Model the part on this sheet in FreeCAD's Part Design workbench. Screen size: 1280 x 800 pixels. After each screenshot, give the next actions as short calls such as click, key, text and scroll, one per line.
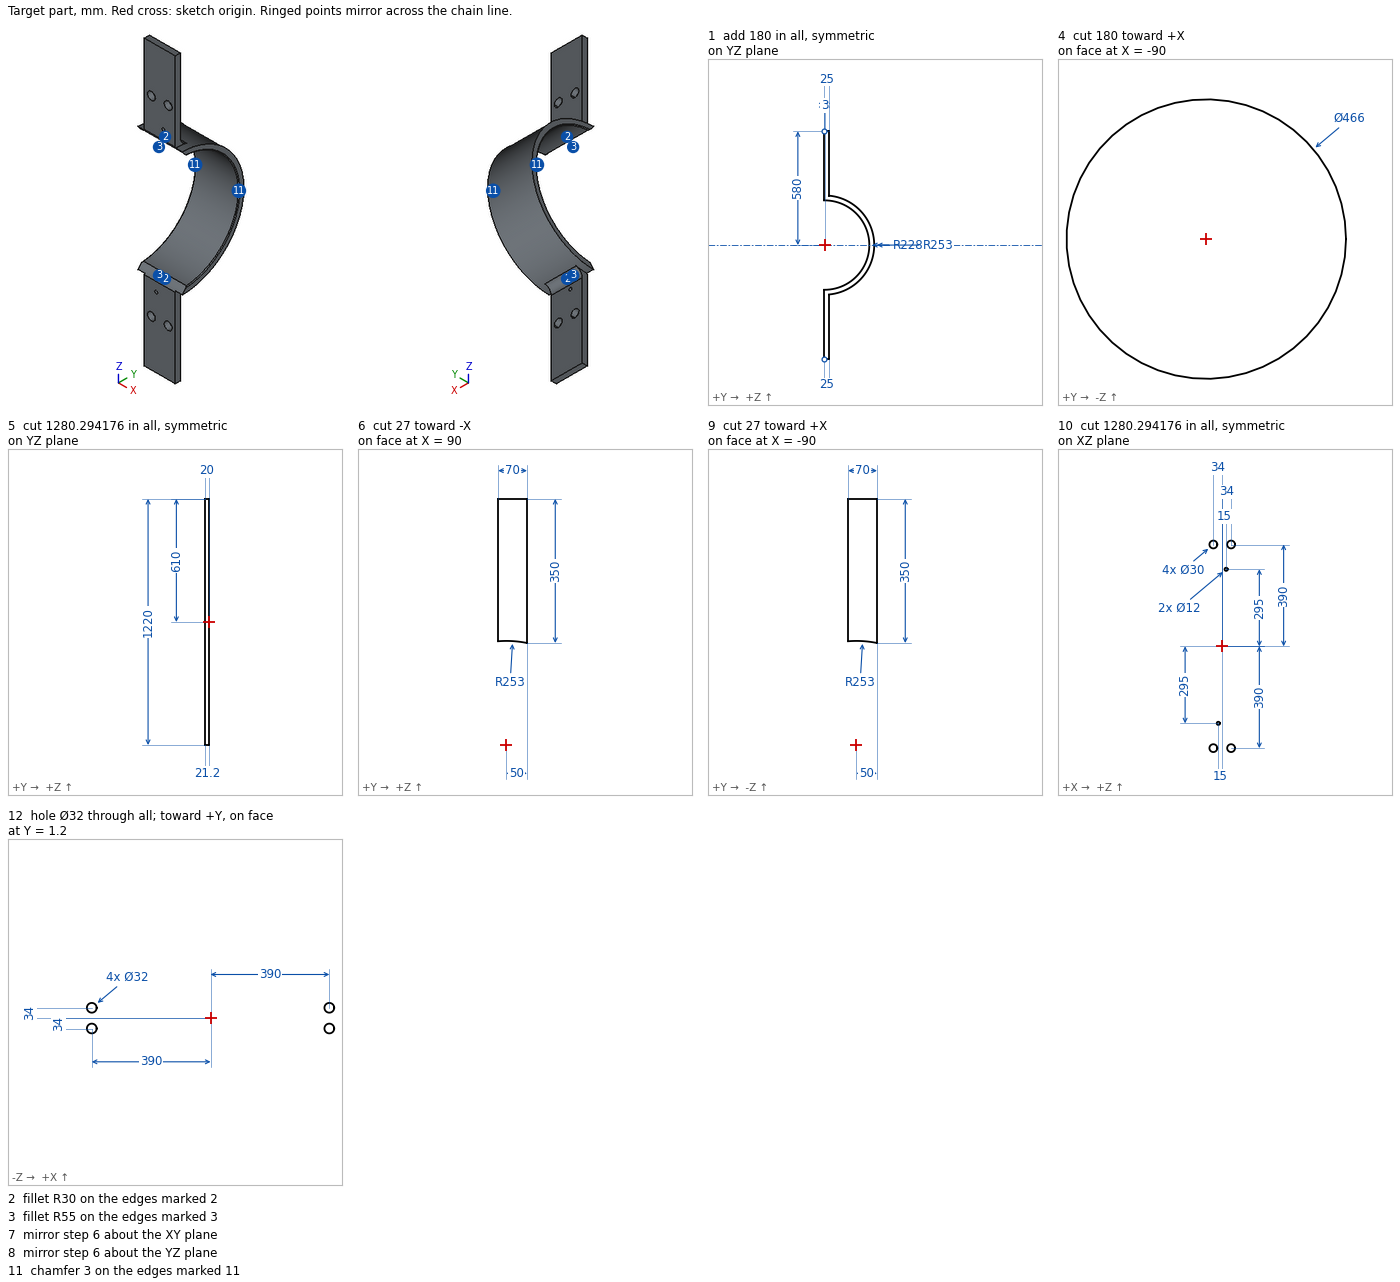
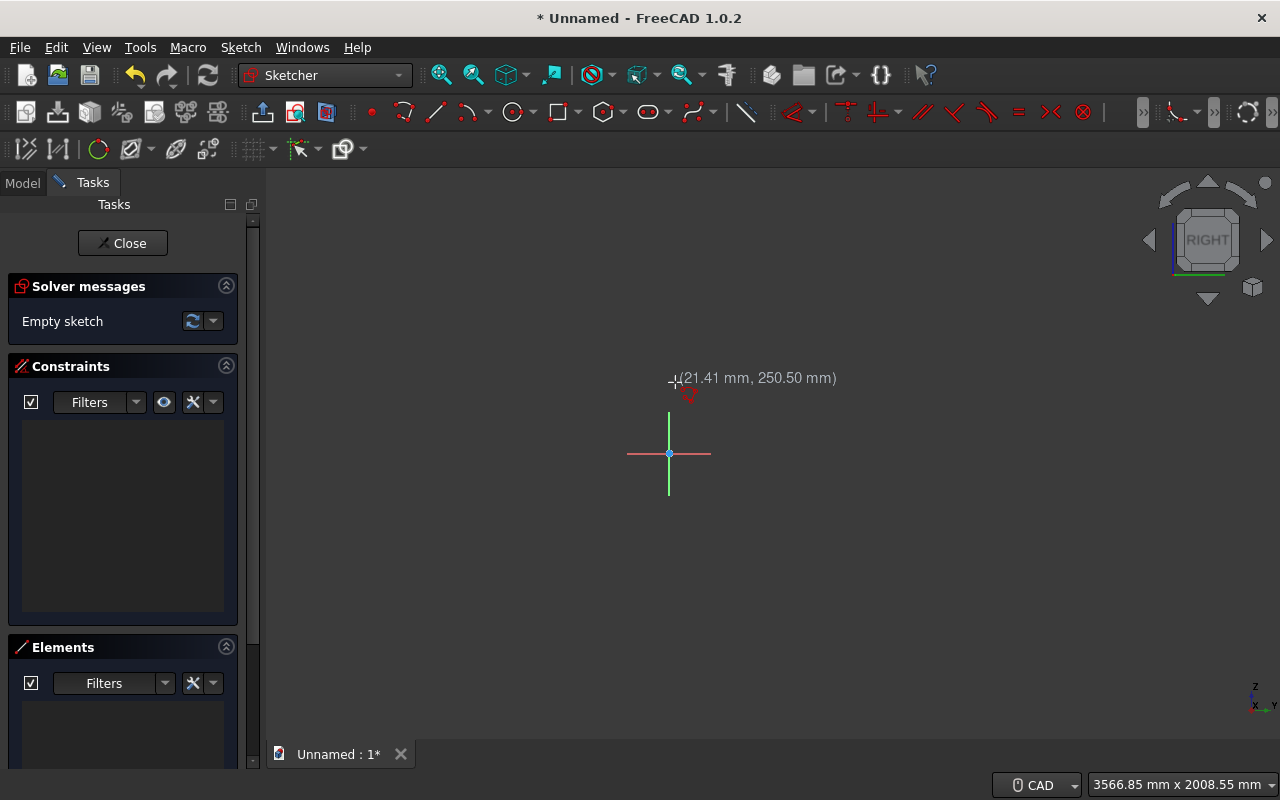
scroll(675, 289, up, 5)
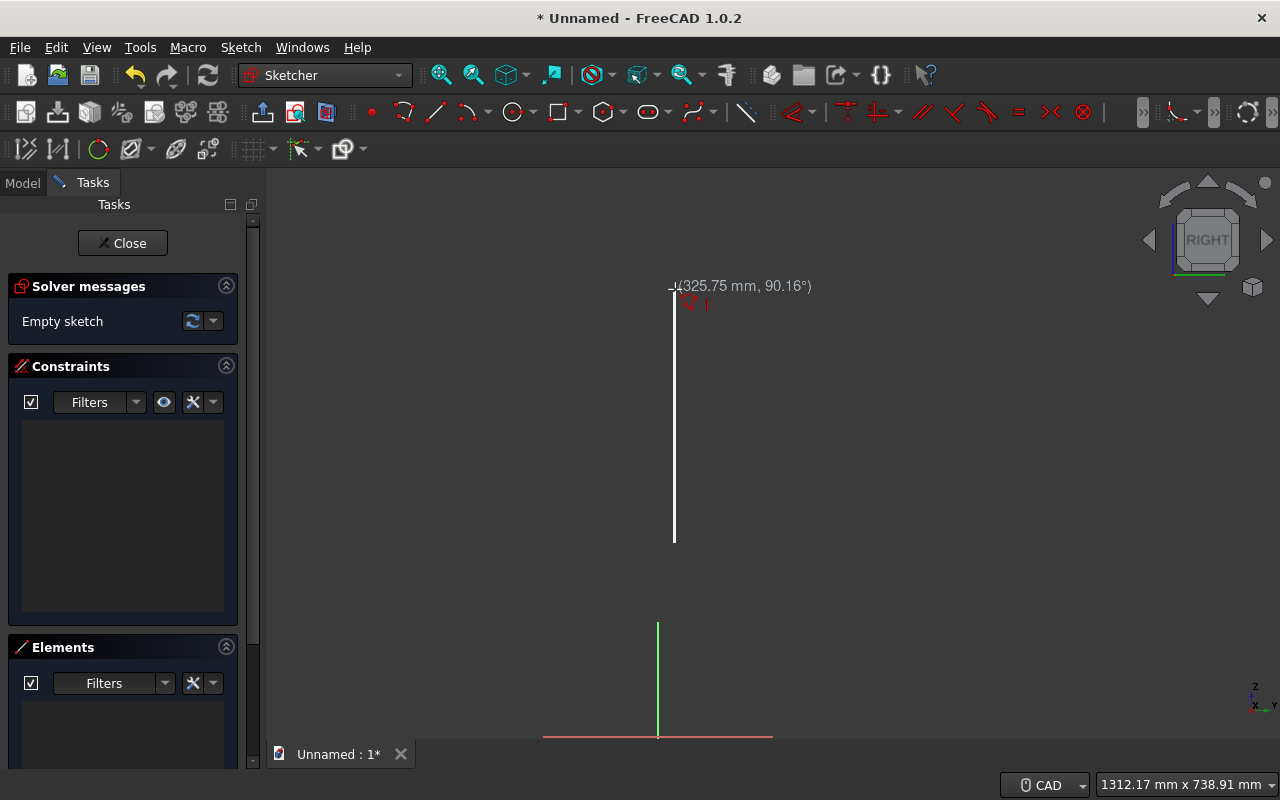
click(675, 288)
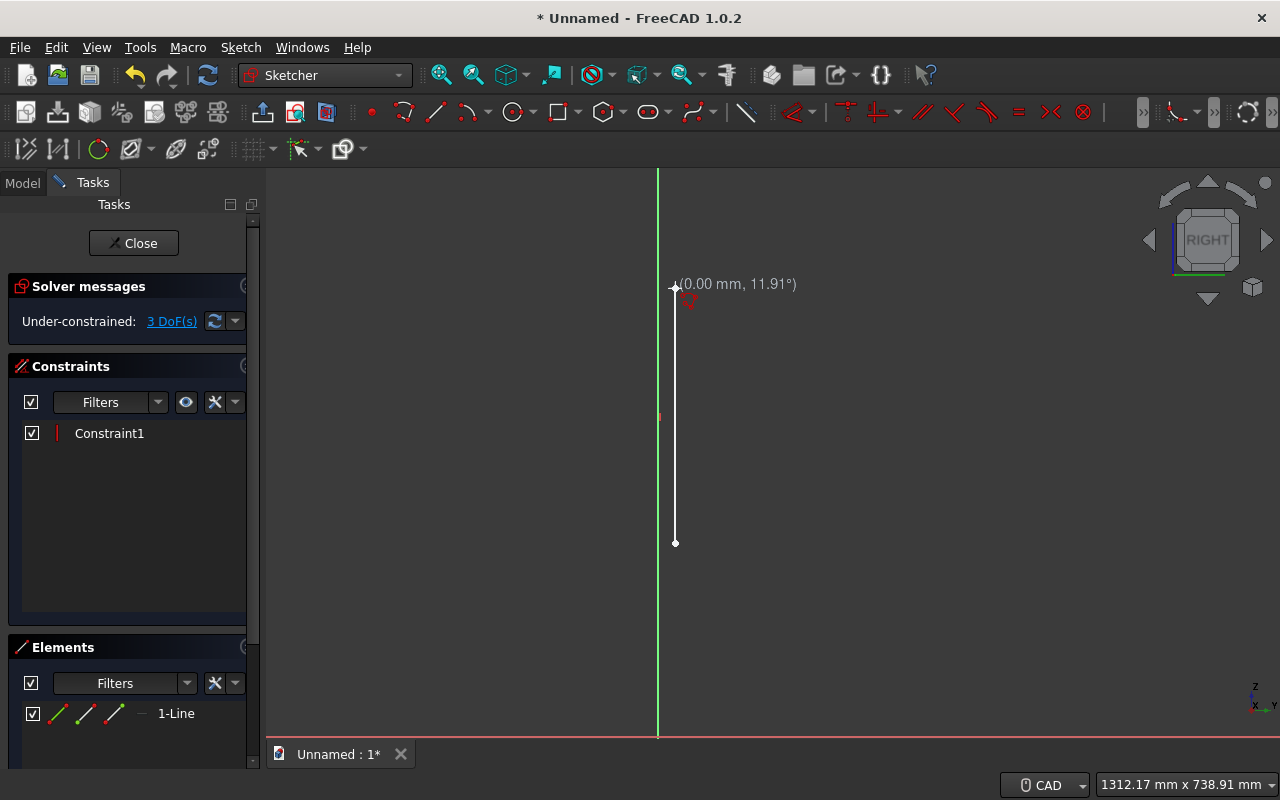
scroll(656, 288, up, 10)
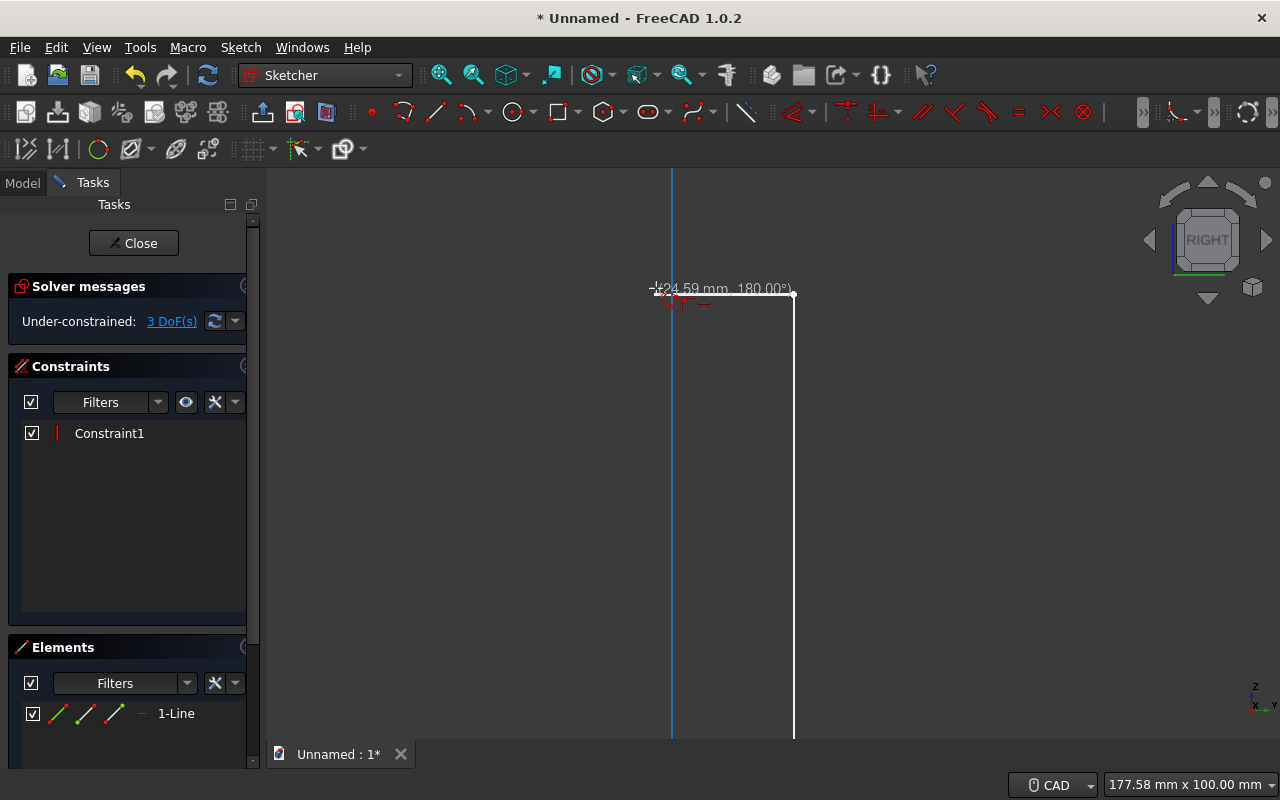
click(655, 287)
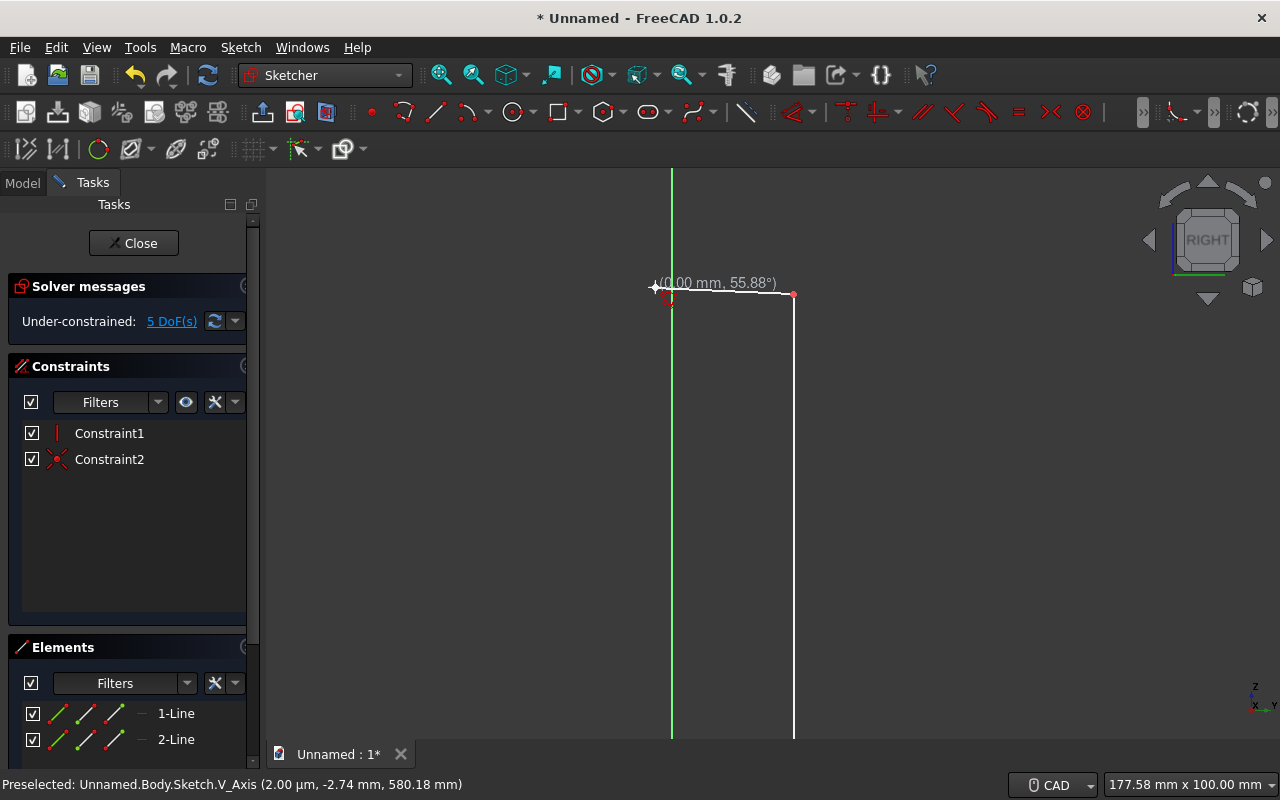
scroll(669, 289, down, 15)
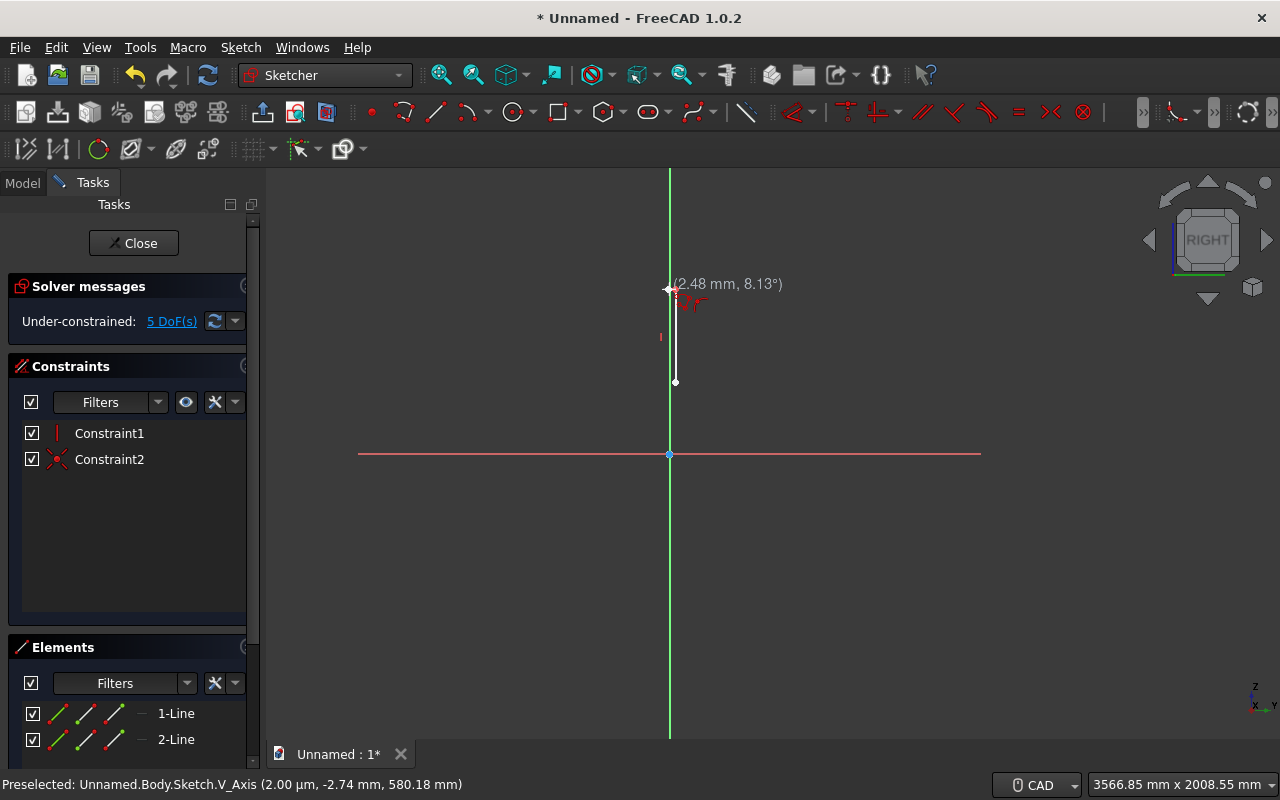
scroll(669, 389, up, 15)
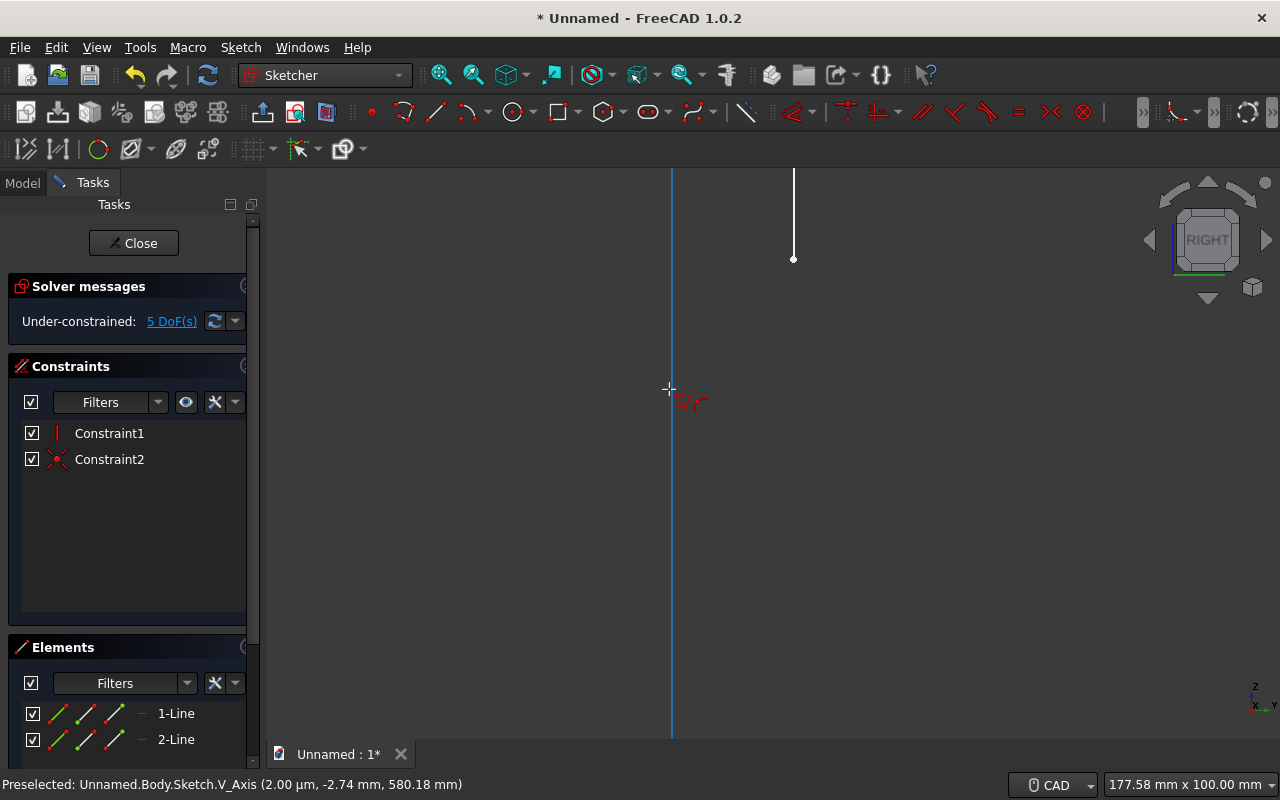
click(655, 388)
right_click(655, 388)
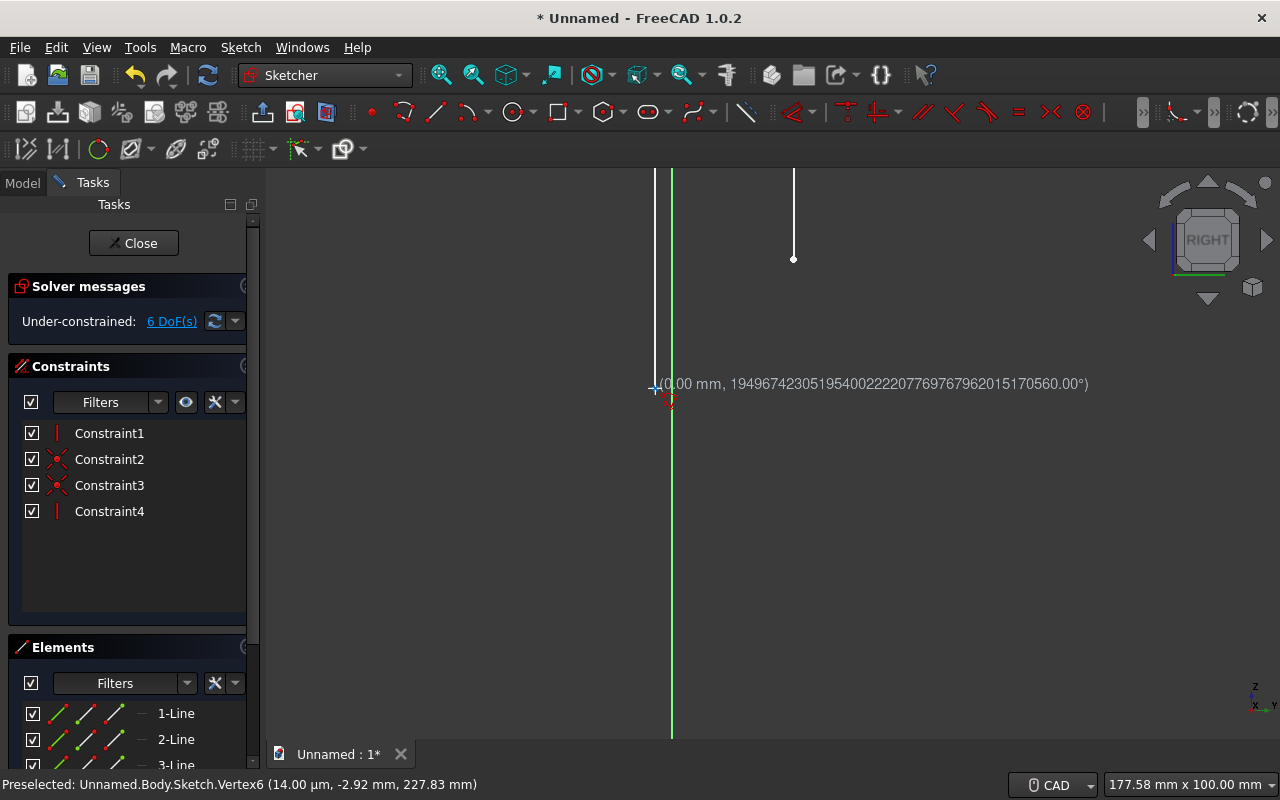
scroll(669, 389, down, 15)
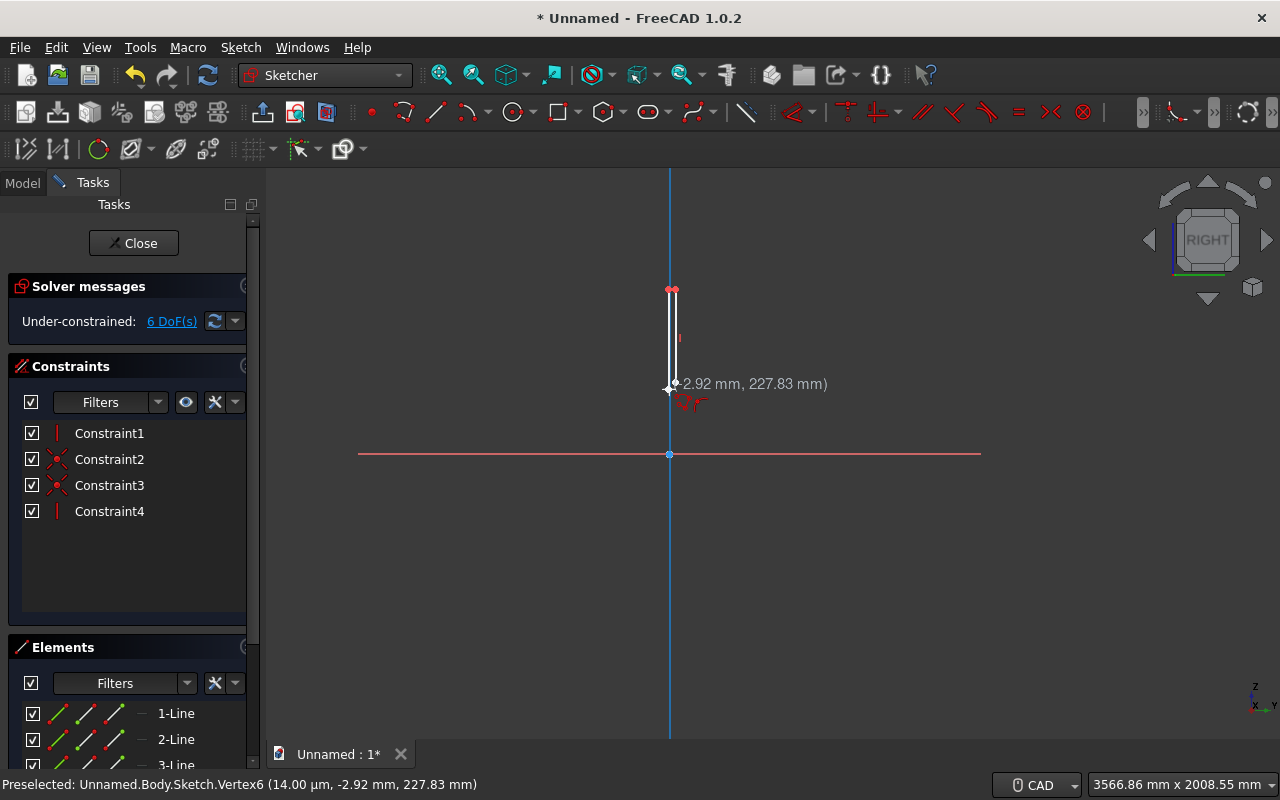
scroll(669, 519, up, 15)